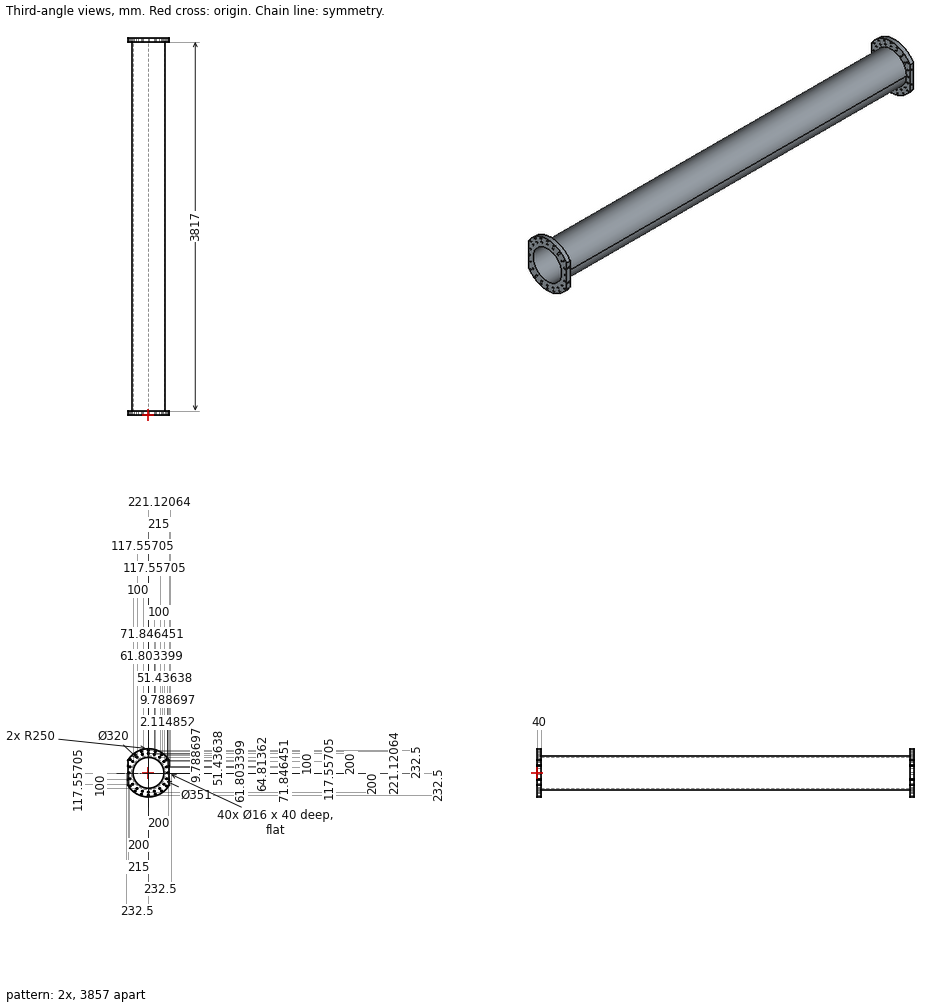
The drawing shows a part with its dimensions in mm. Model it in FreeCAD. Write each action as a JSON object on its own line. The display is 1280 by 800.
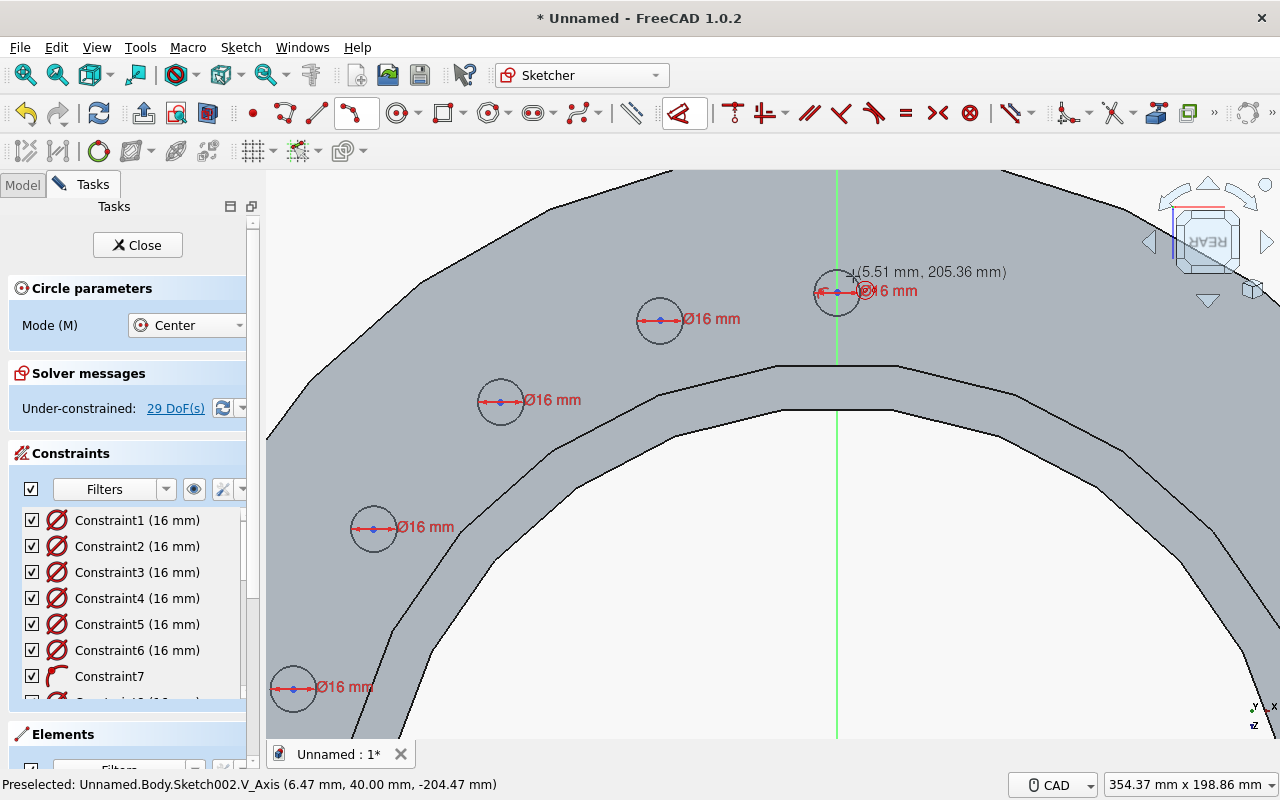
{"action": "left_click", "coordinate": [1014, 320]}
{"action": "mouse_move", "coordinate": [1030, 304]}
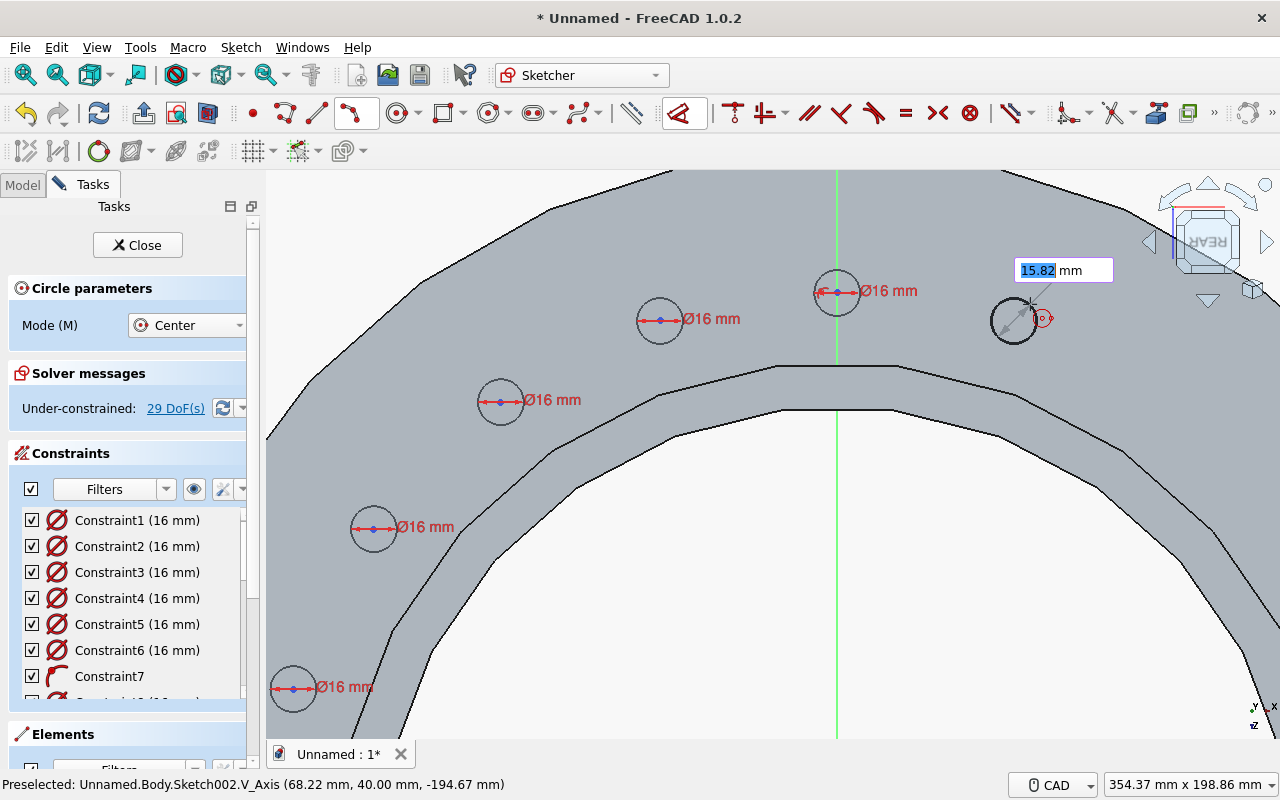
{"action": "type", "text": "16"}
{"action": "key", "text": "Return"}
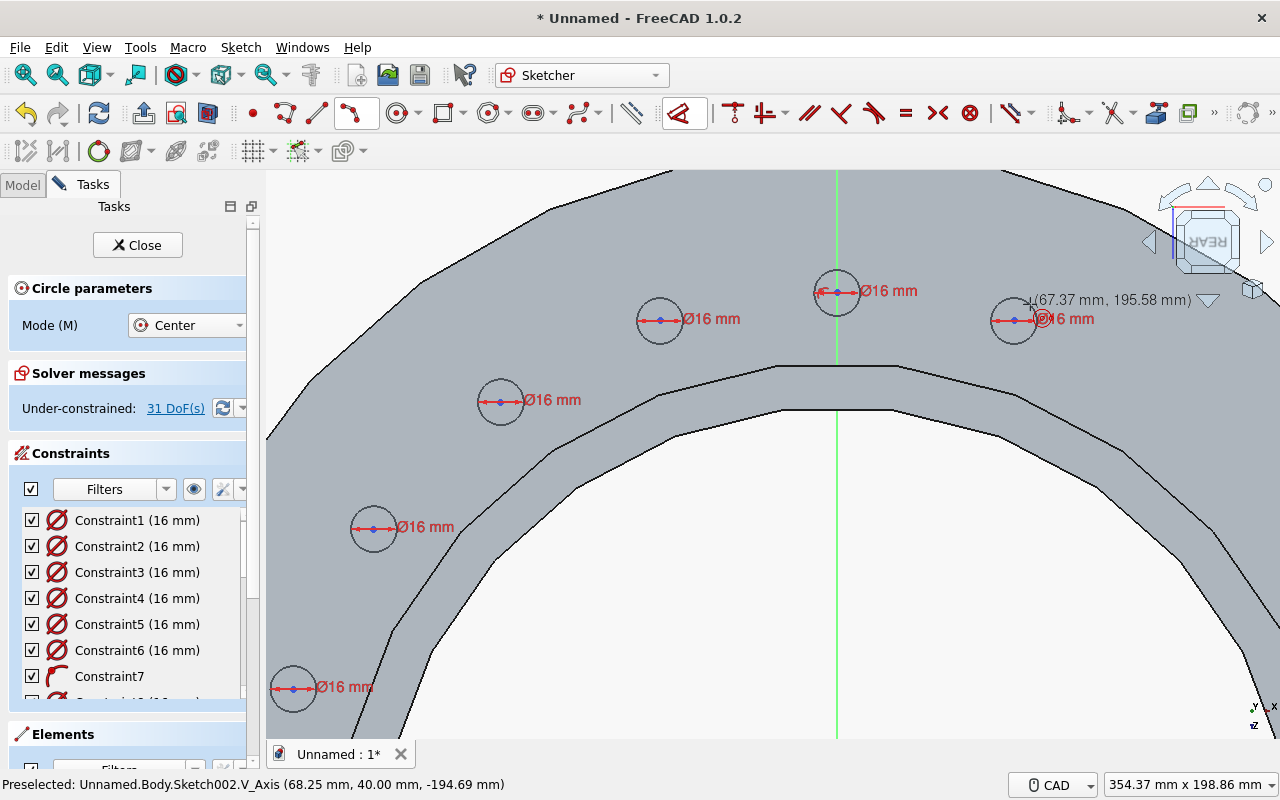
{"action": "scroll", "coordinate": [661, 320], "scroll_direction": "down", "scroll_amount": 7}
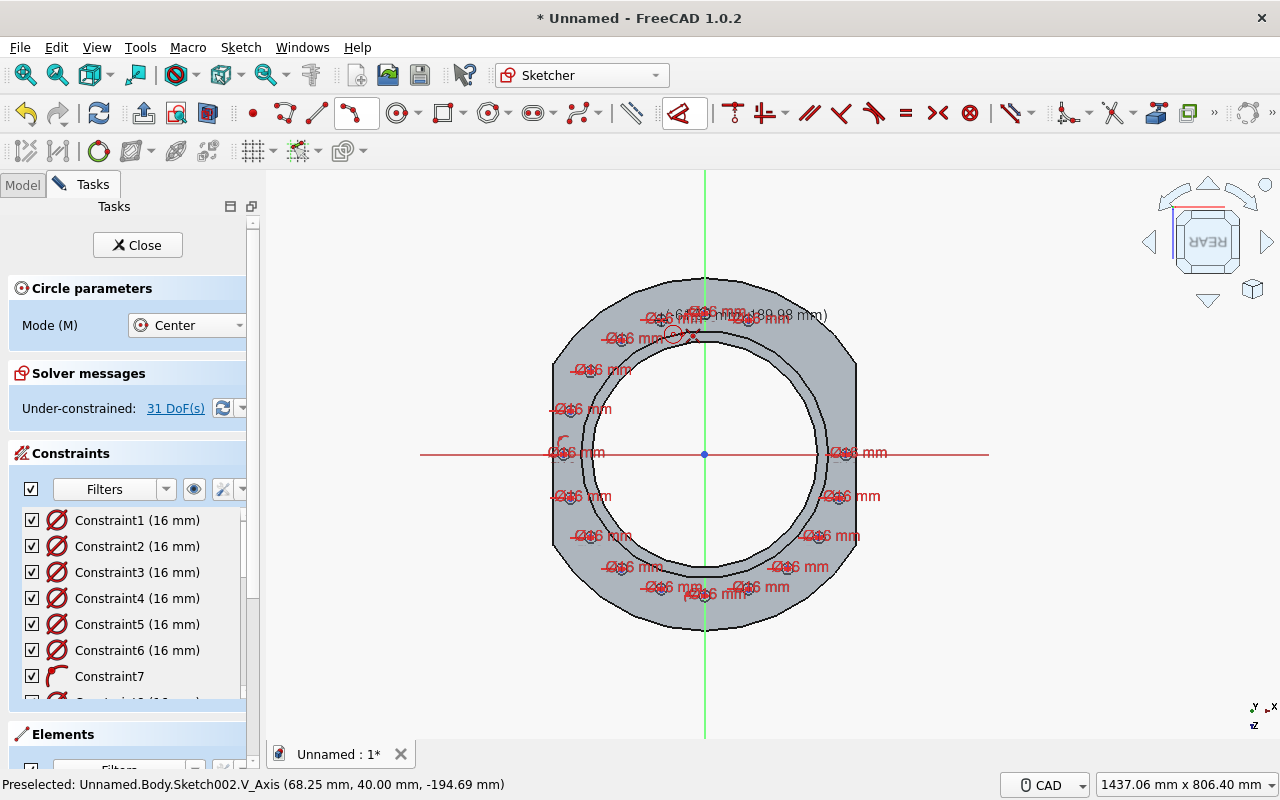
{"action": "scroll", "coordinate": [788, 340], "scroll_direction": "up", "scroll_amount": 7}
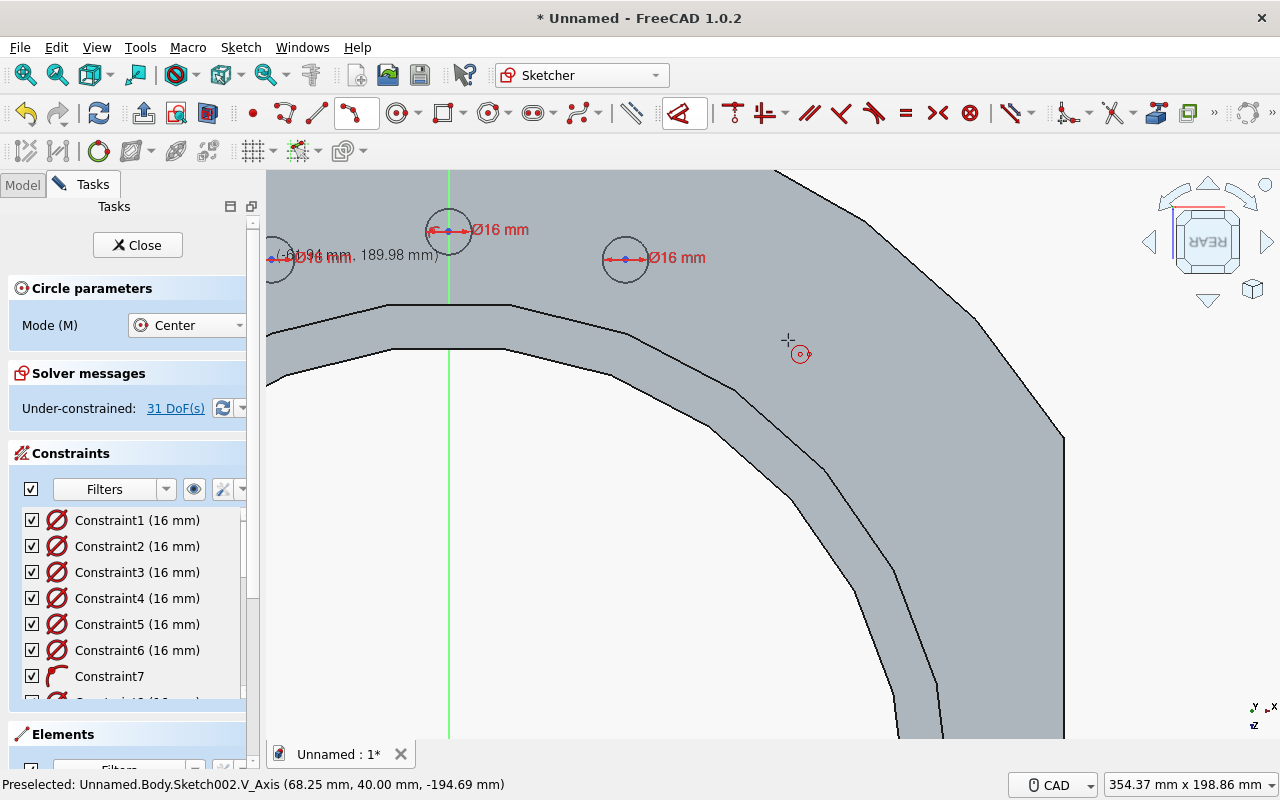
{"action": "left_click", "coordinate": [785, 340]}
{"action": "mouse_move", "coordinate": [801, 324]}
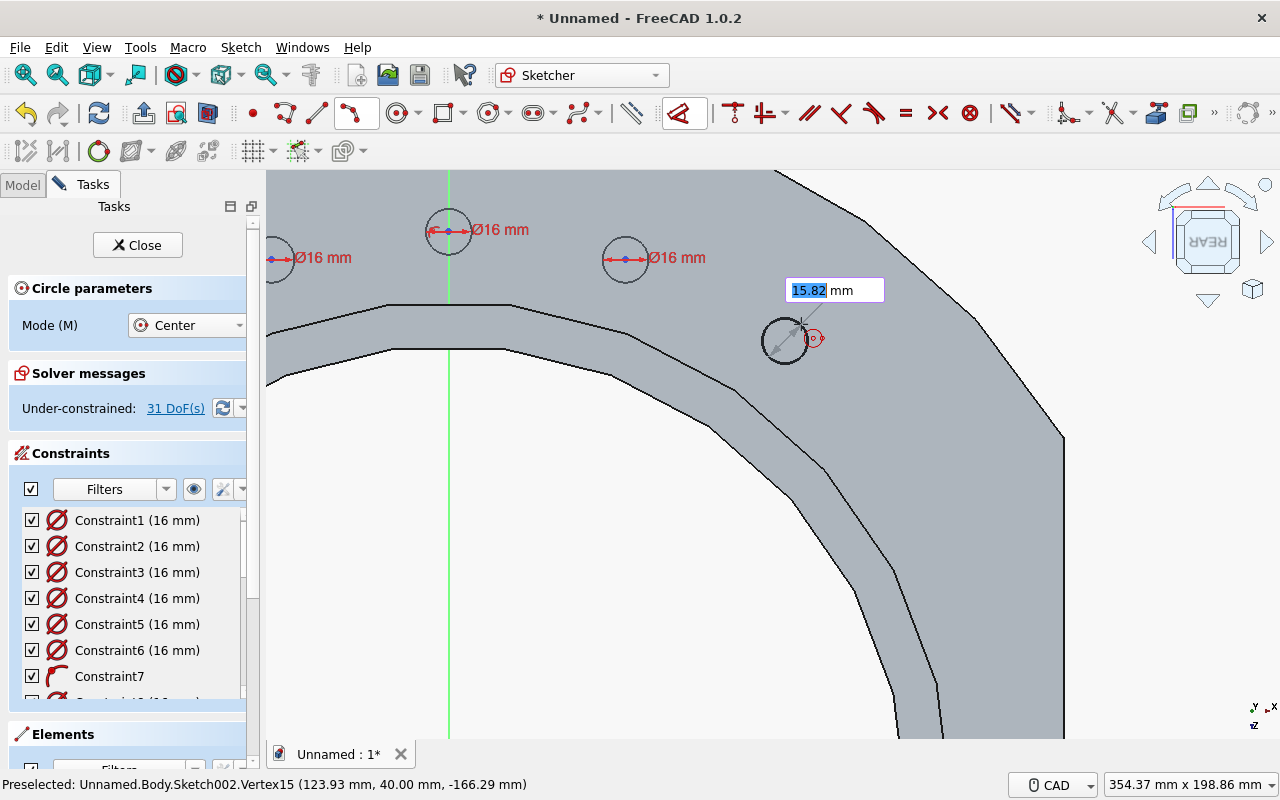
{"action": "type", "text": "16"}
{"action": "key", "text": "Return"}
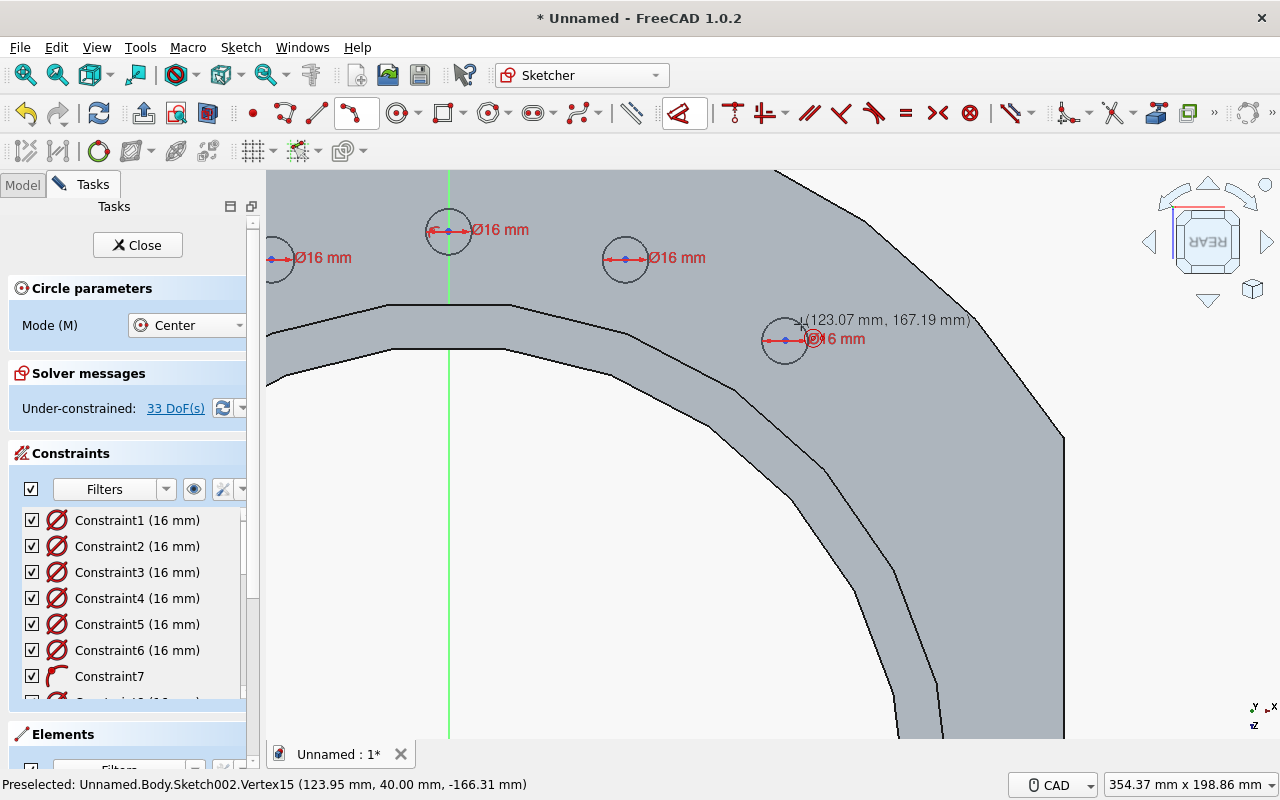
{"action": "left_click", "coordinate": [912, 467]}
{"action": "mouse_move", "coordinate": [928, 451]}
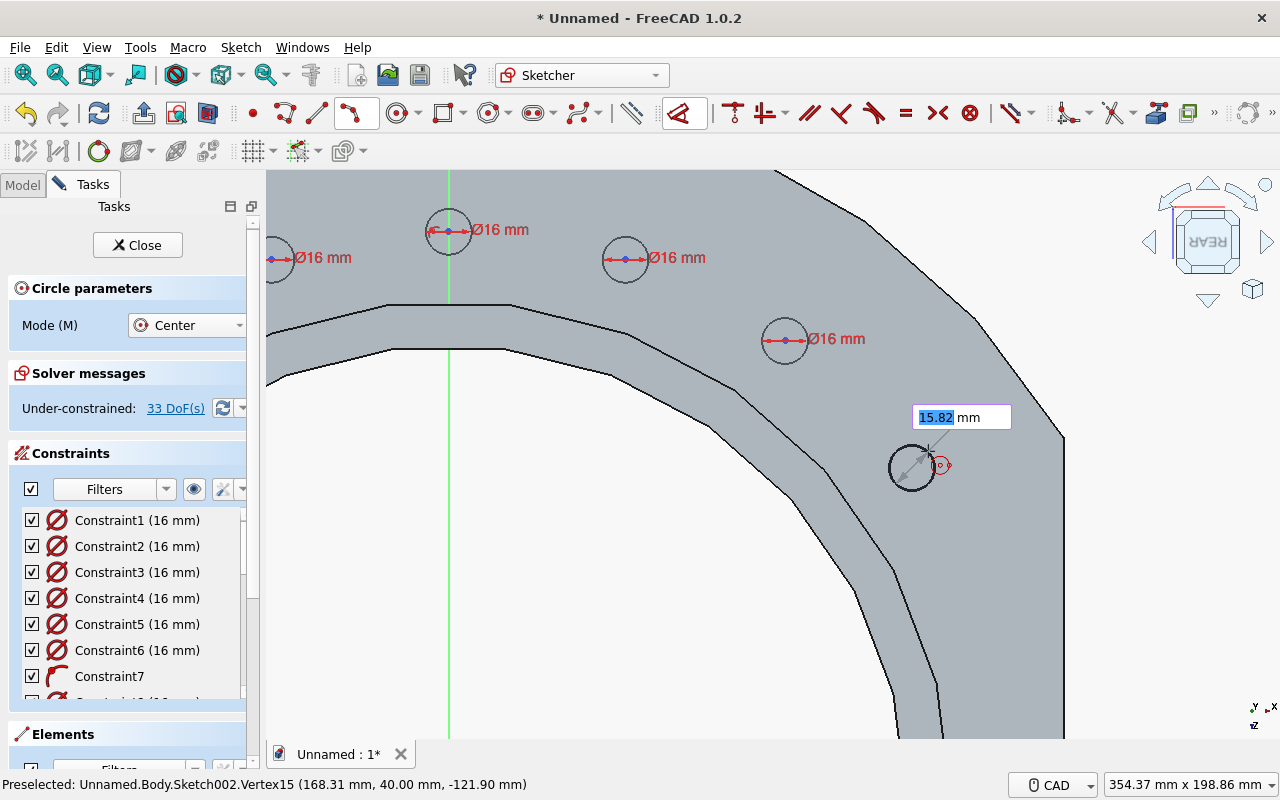
{"action": "type", "text": "16"}
{"action": "key", "text": "Return"}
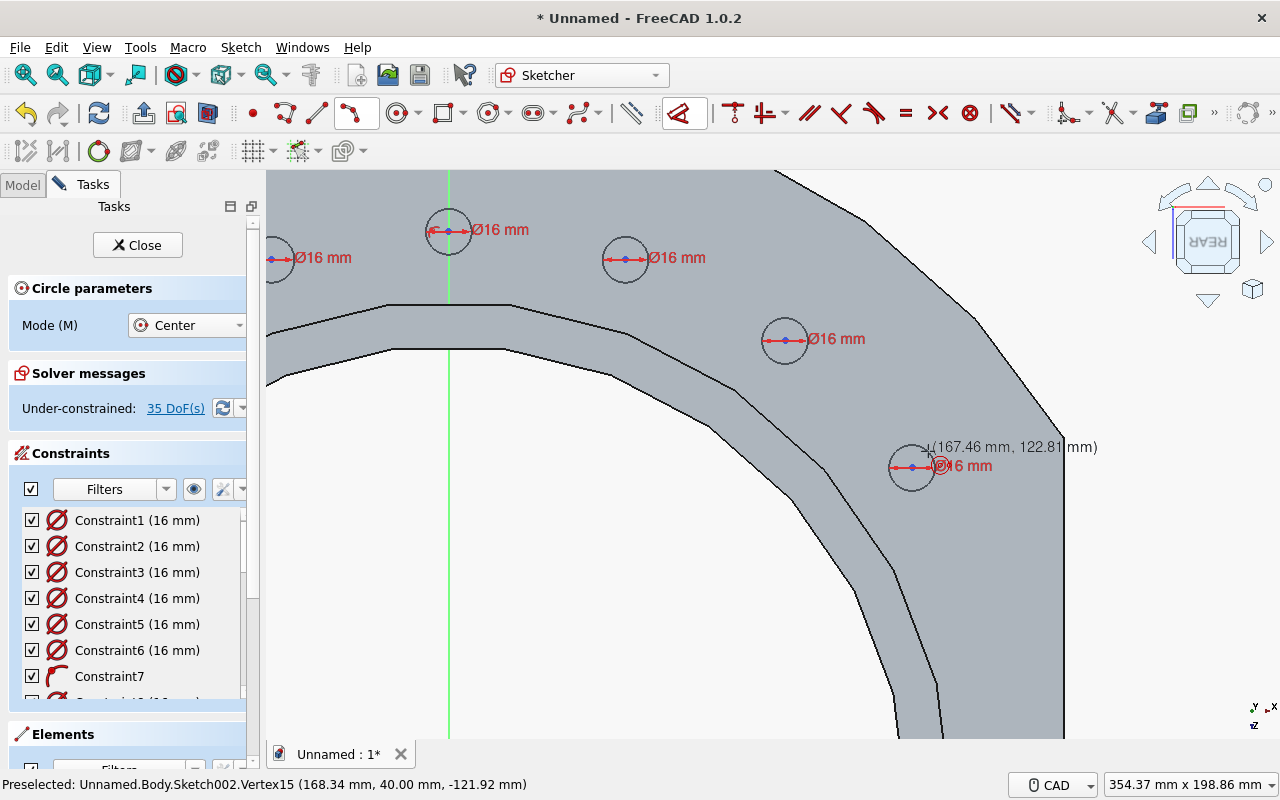
{"action": "left_click", "coordinate": [993, 627]}
{"action": "mouse_move", "coordinate": [1009, 610]}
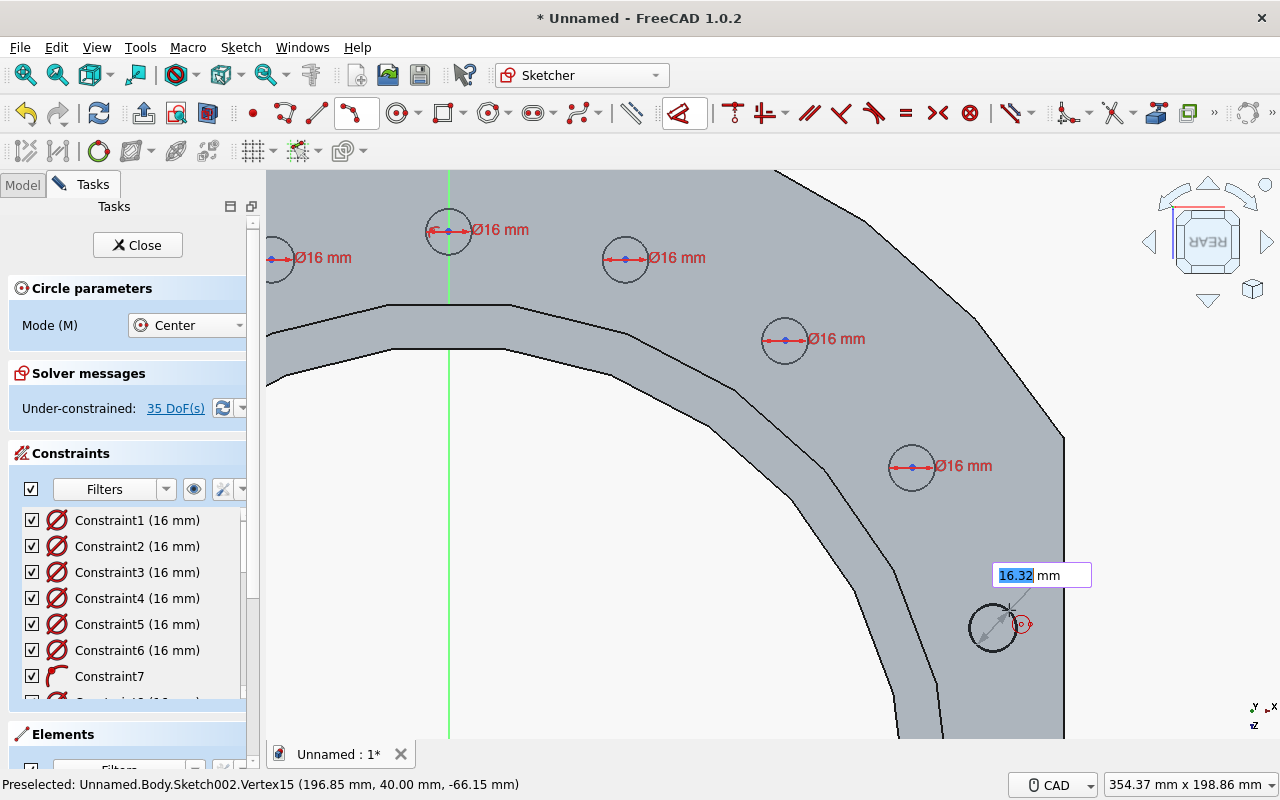
{"action": "type", "text": "16"}
{"action": "key", "text": "Return"}